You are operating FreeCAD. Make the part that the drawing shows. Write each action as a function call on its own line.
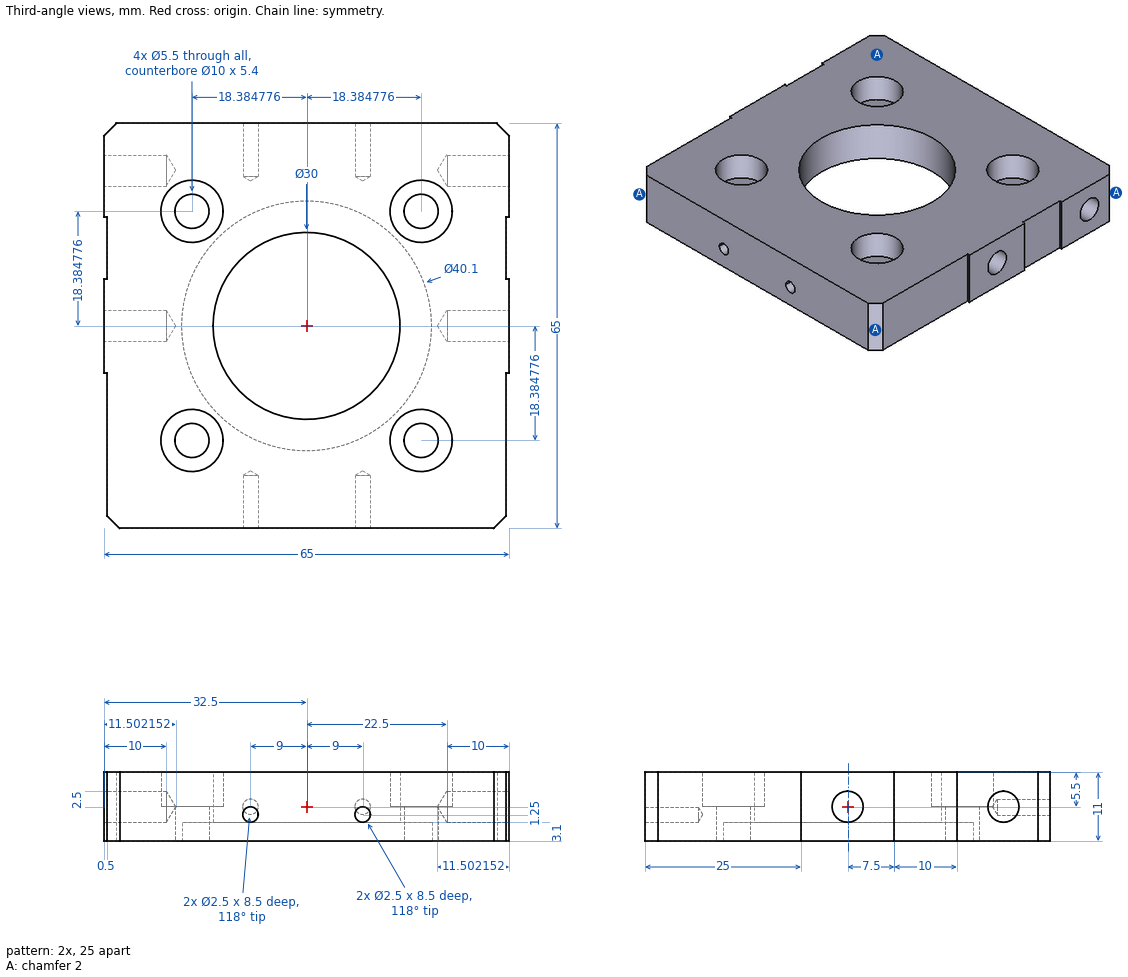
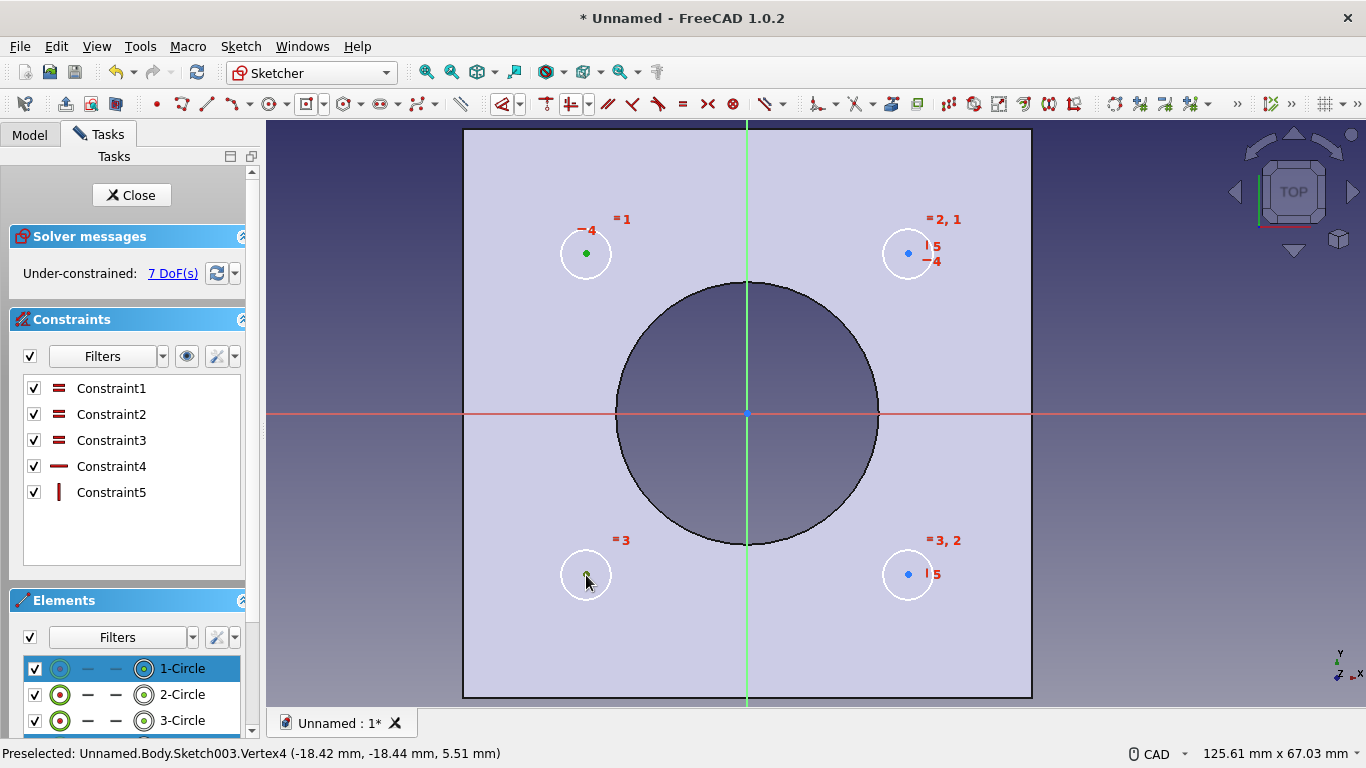
click(588, 104)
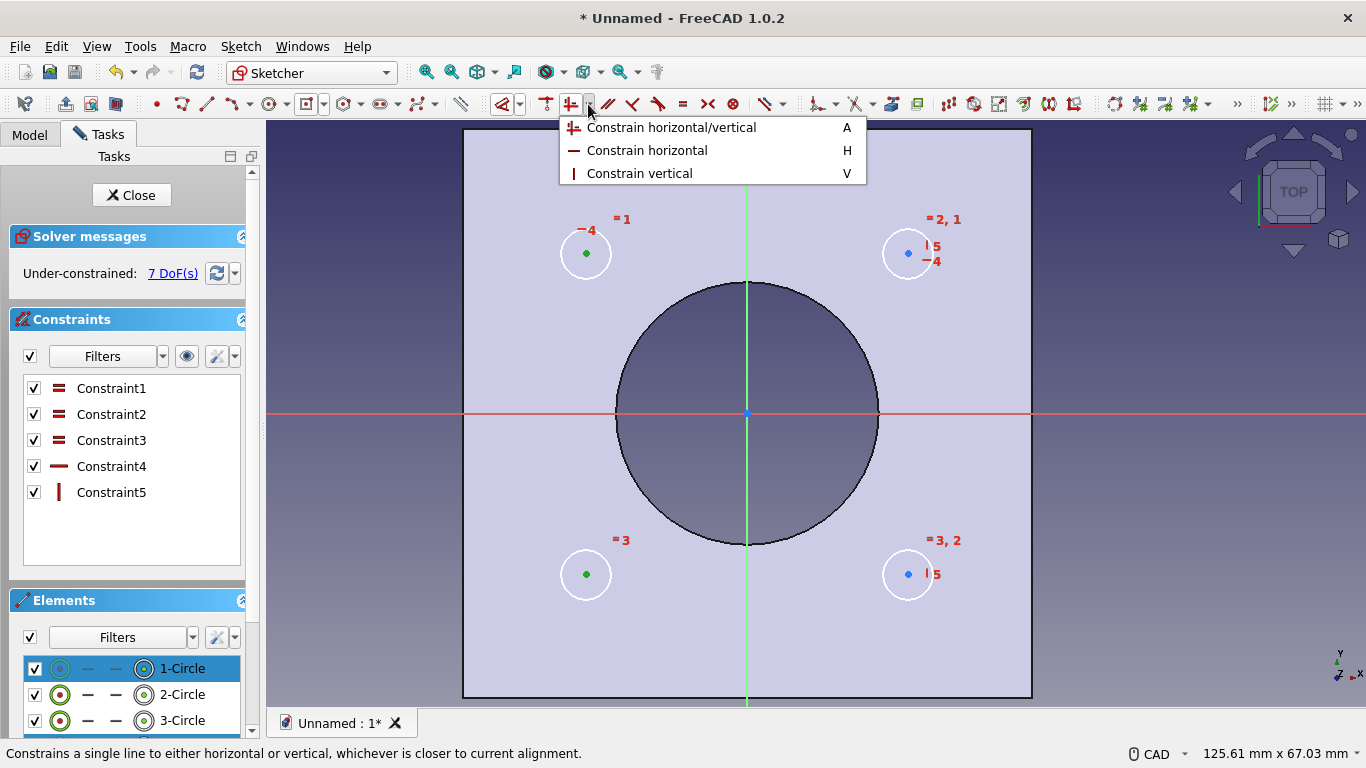
click(713, 174)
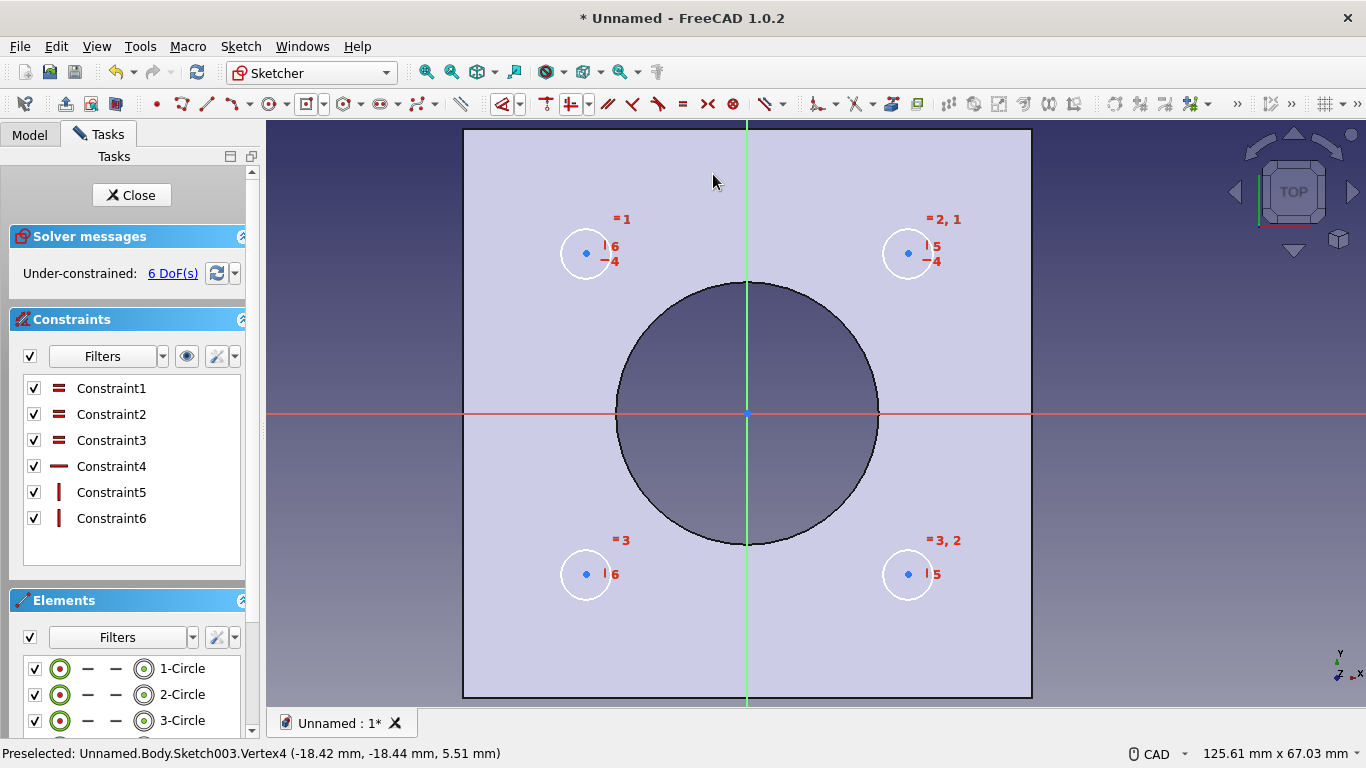
click(908, 575)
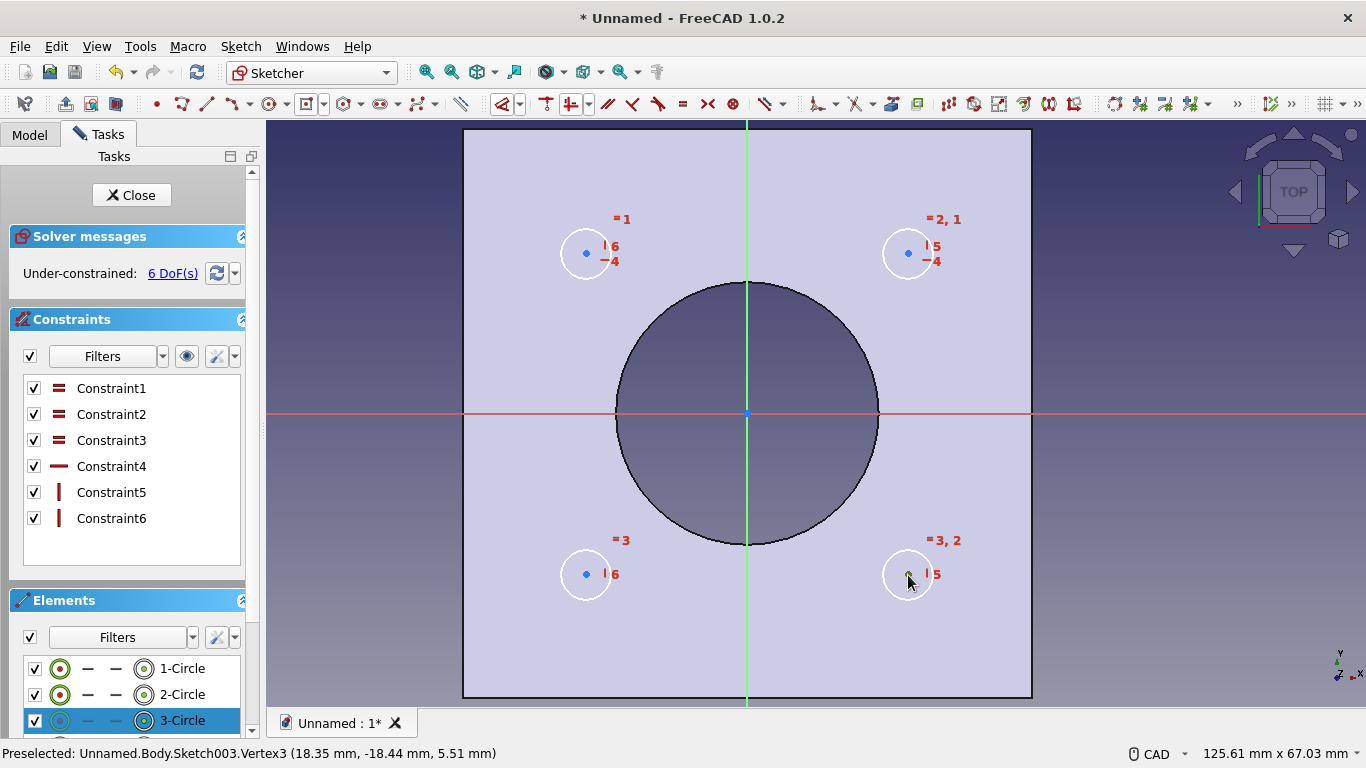
click(586, 575)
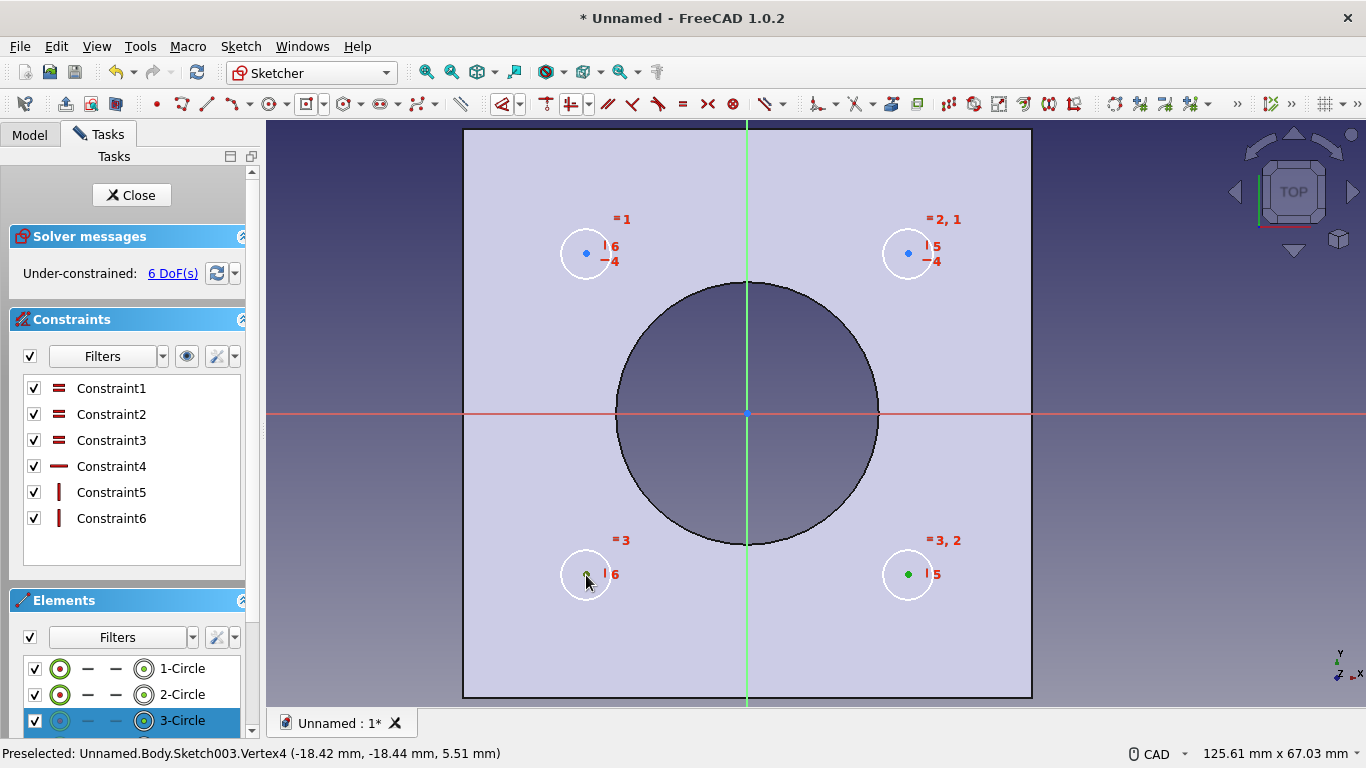
click(588, 104)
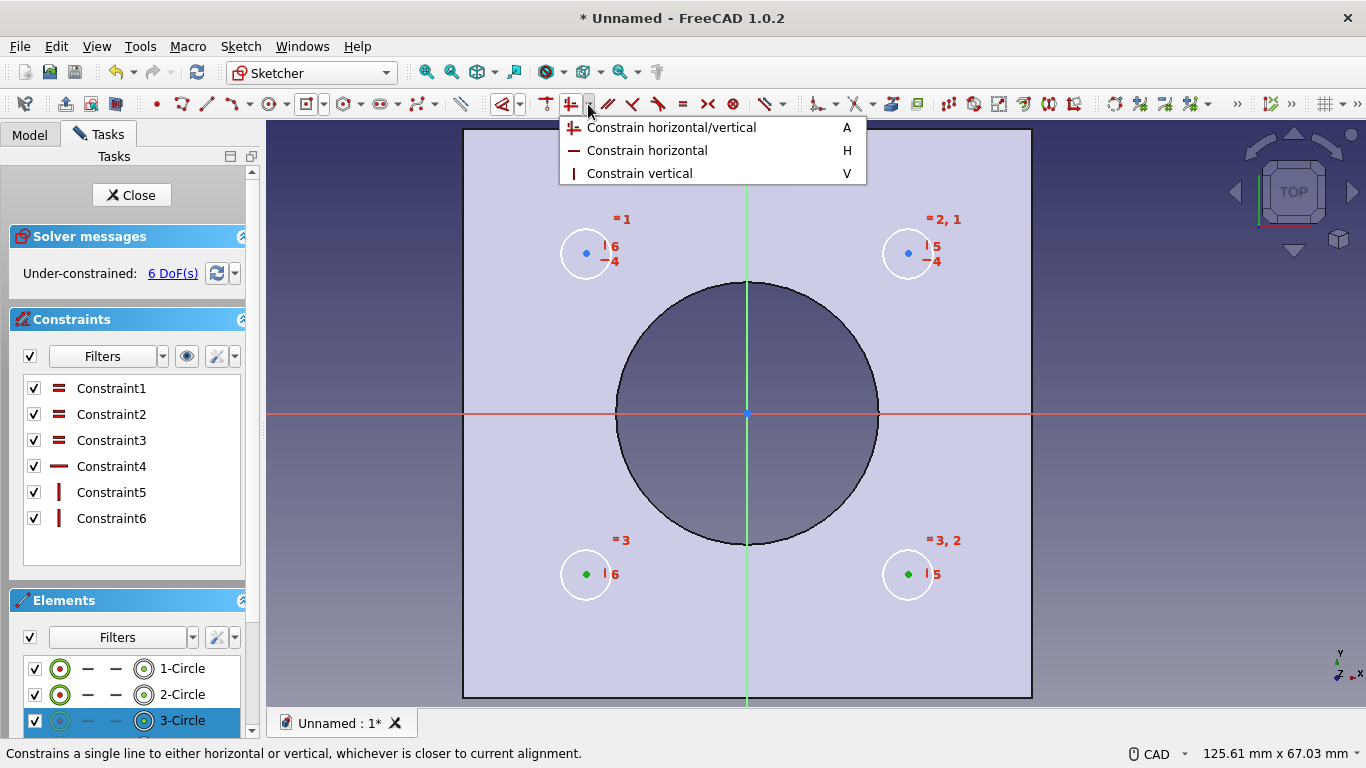
click(713, 150)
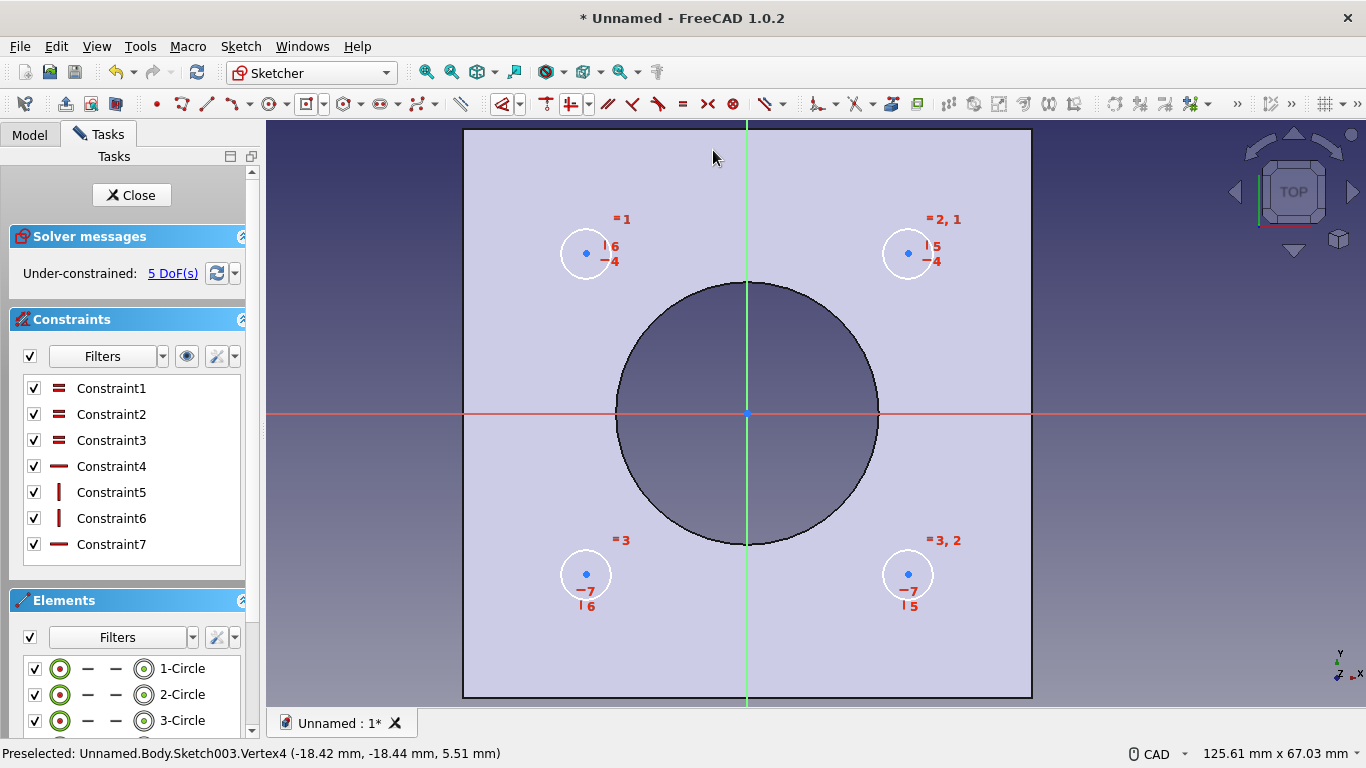
click(603, 236)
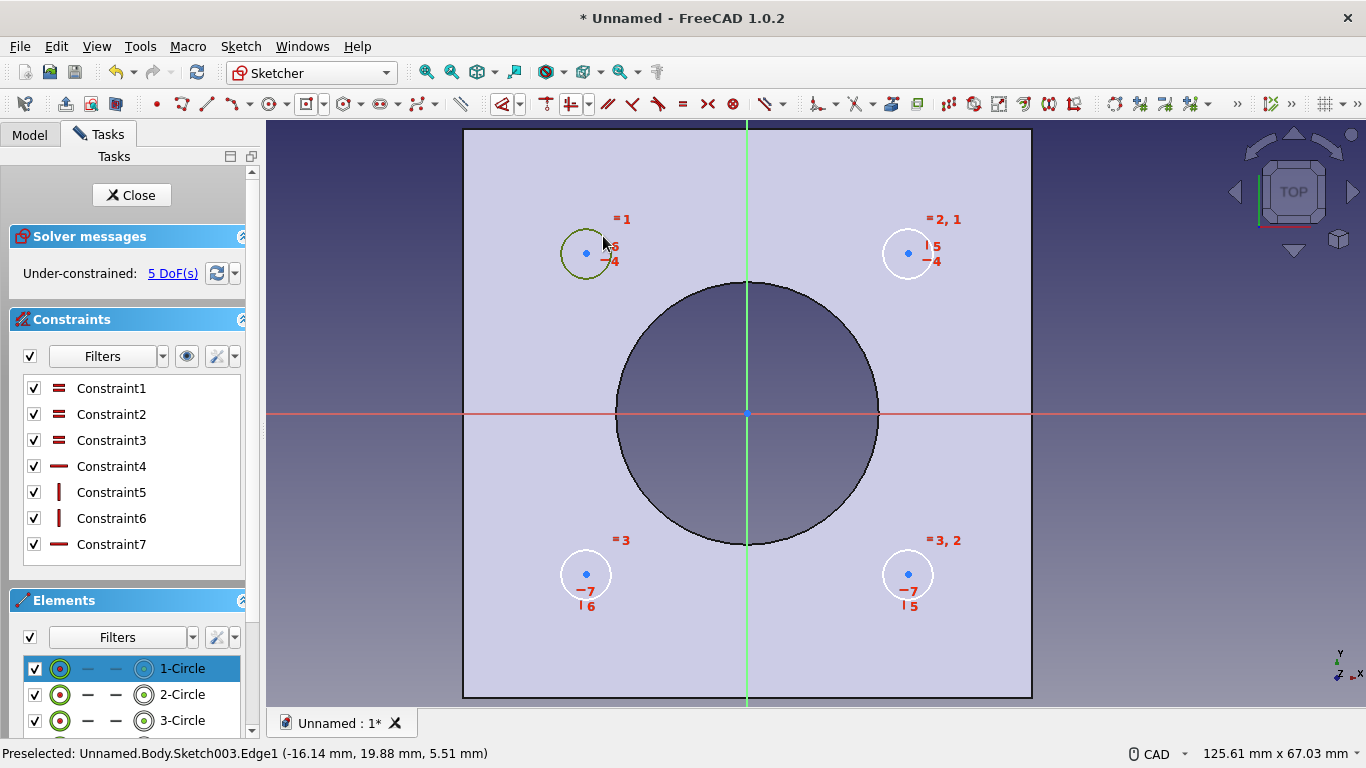
click(520, 104)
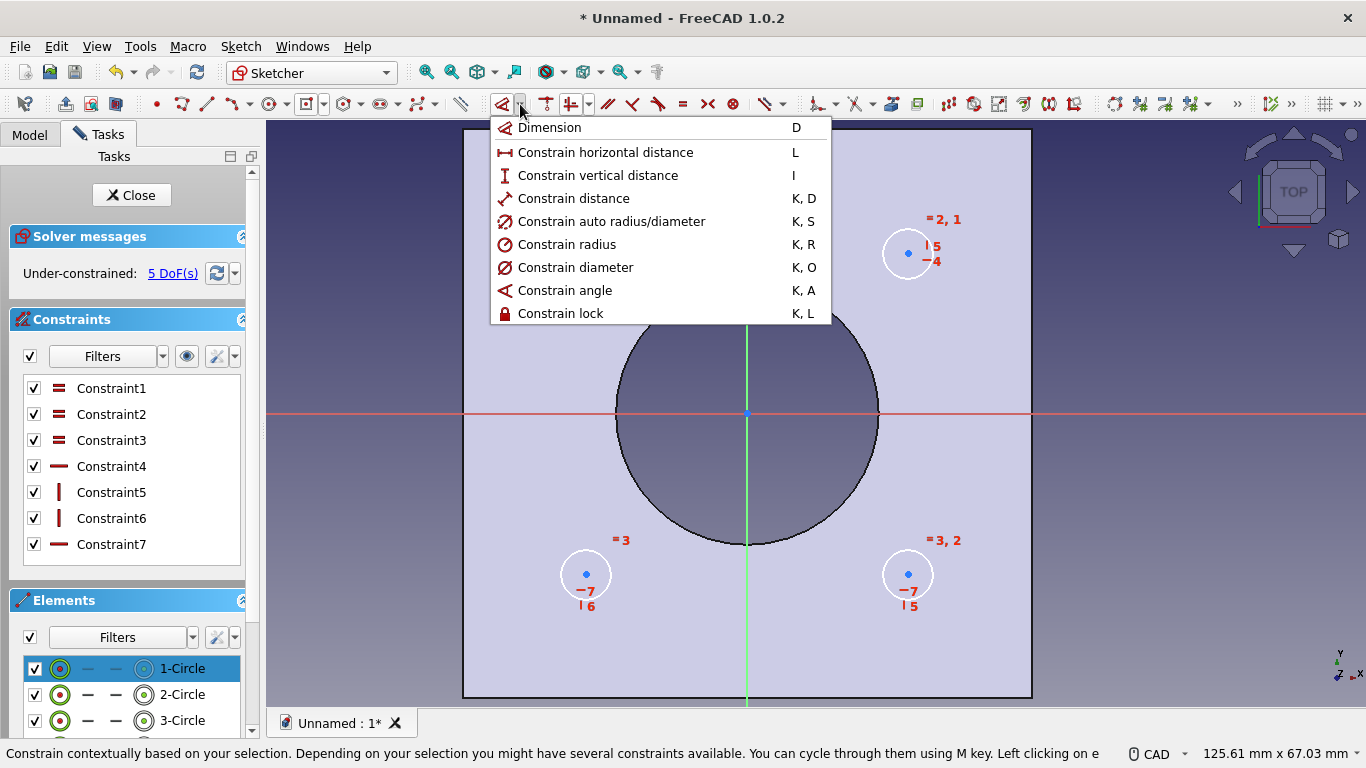
click(661, 268)